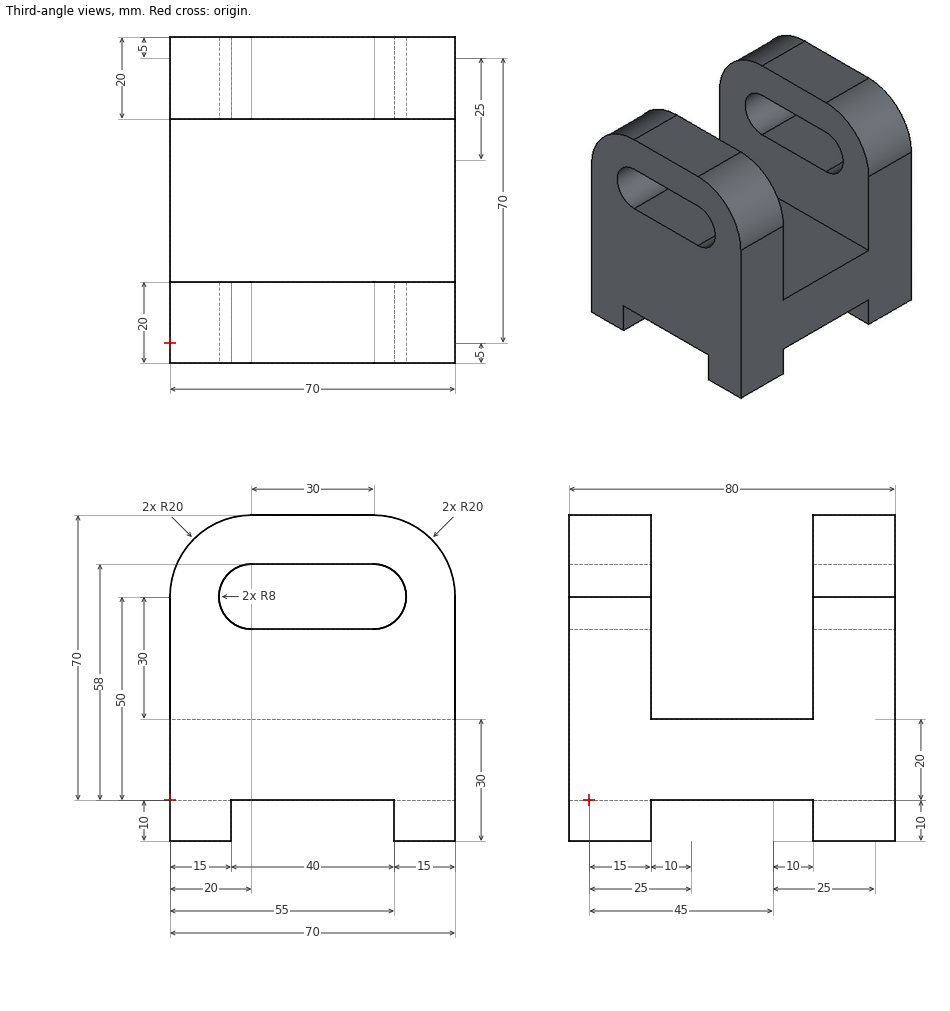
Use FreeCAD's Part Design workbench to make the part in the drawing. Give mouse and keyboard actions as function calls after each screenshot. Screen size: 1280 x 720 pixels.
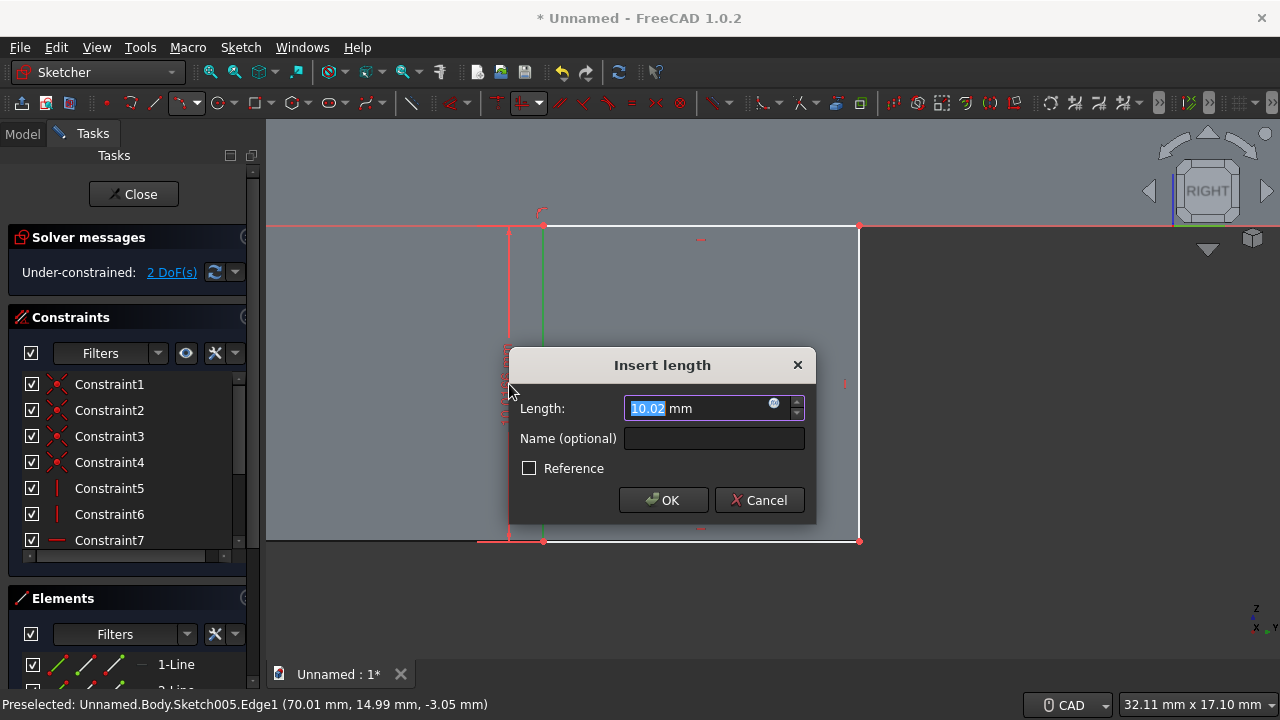
text(10)
key(Return)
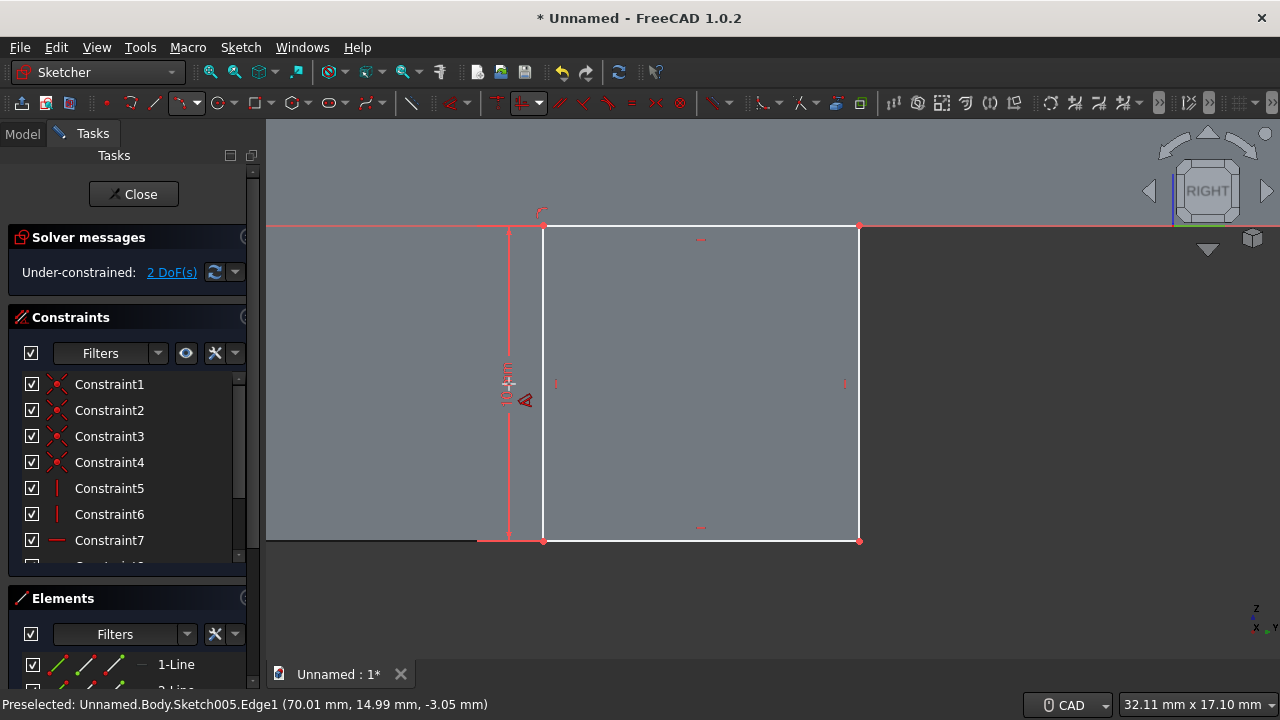
click(638, 541)
click(701, 575)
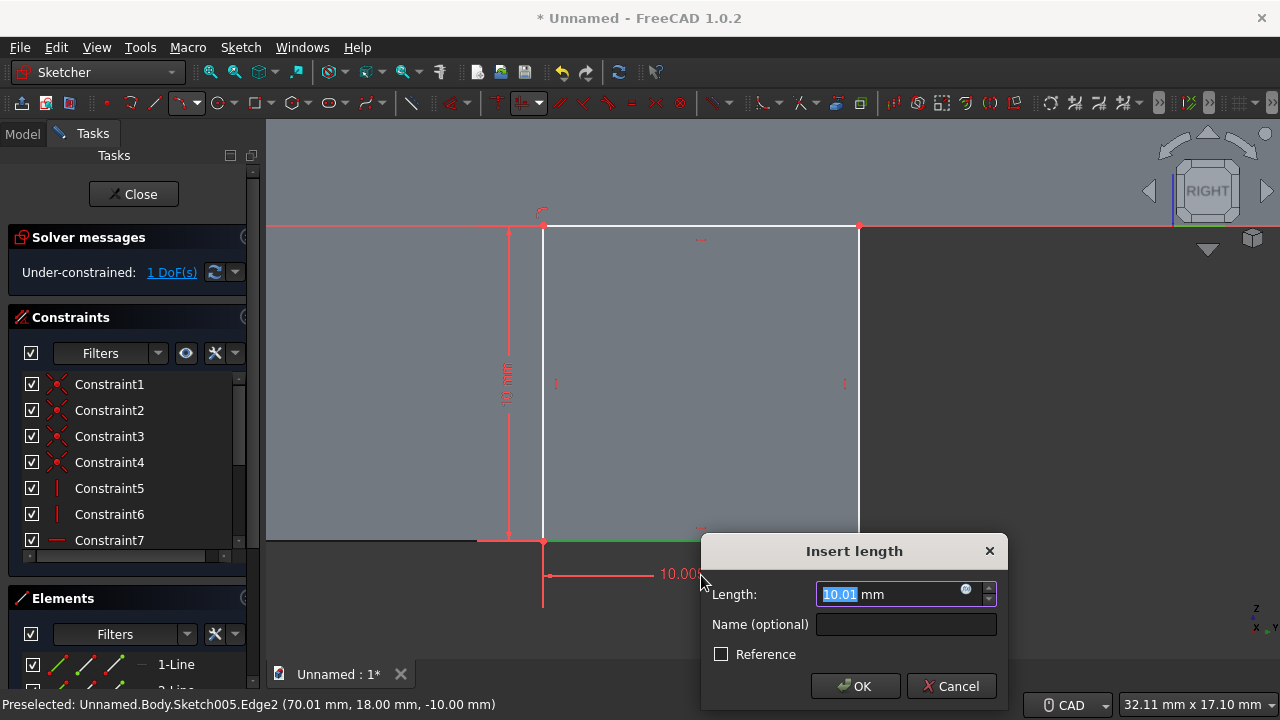
text(10)
key(Return)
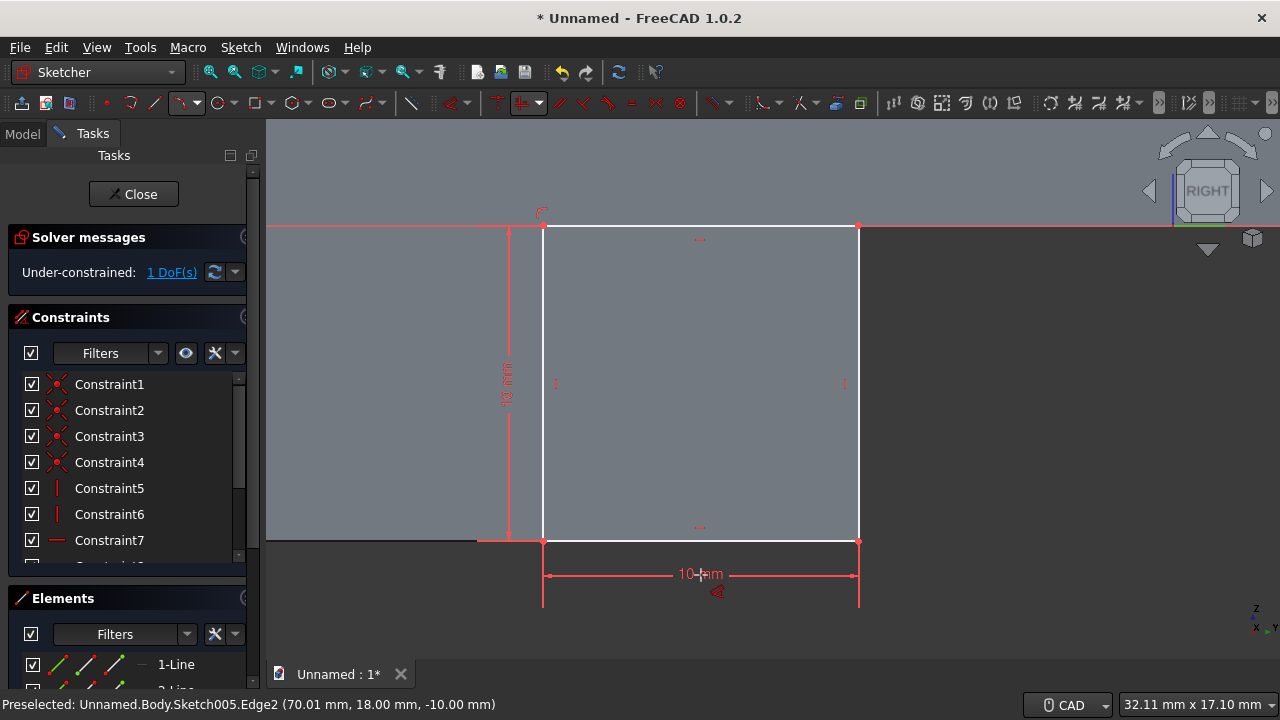
click(543, 226)
click(418, 192)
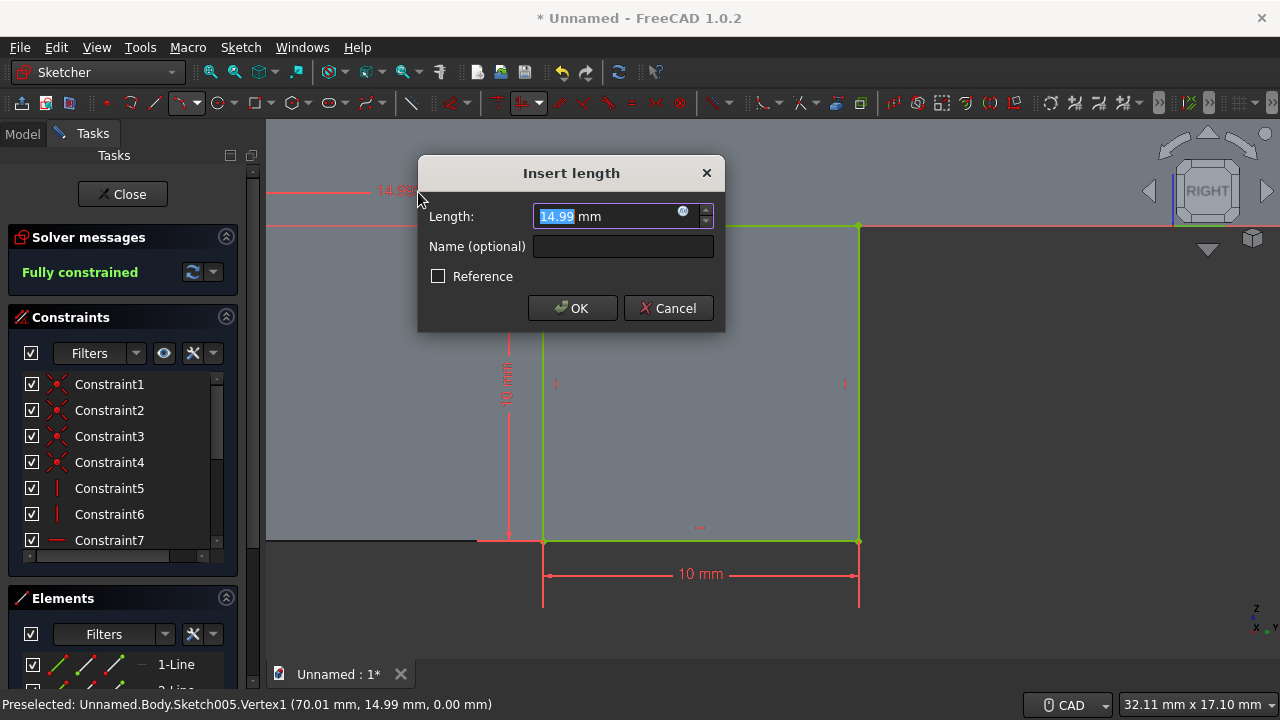
text(15)
key(Return)
key(Escape)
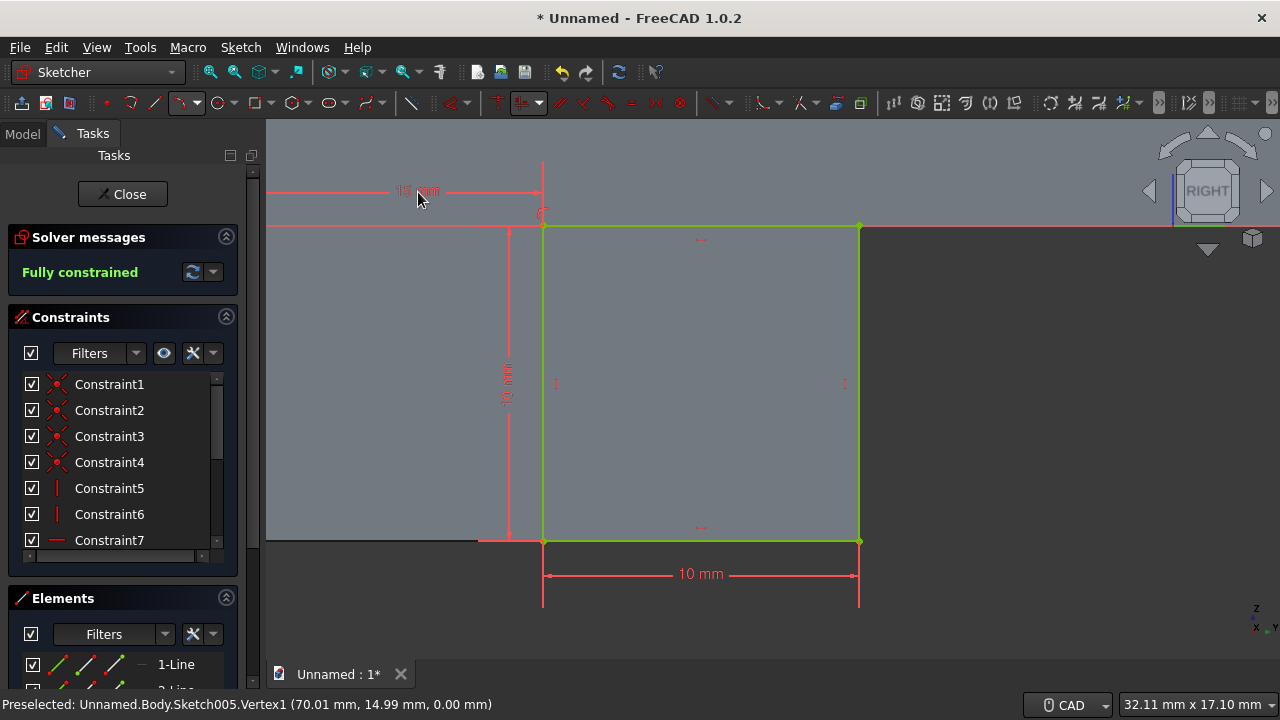
click(123, 194)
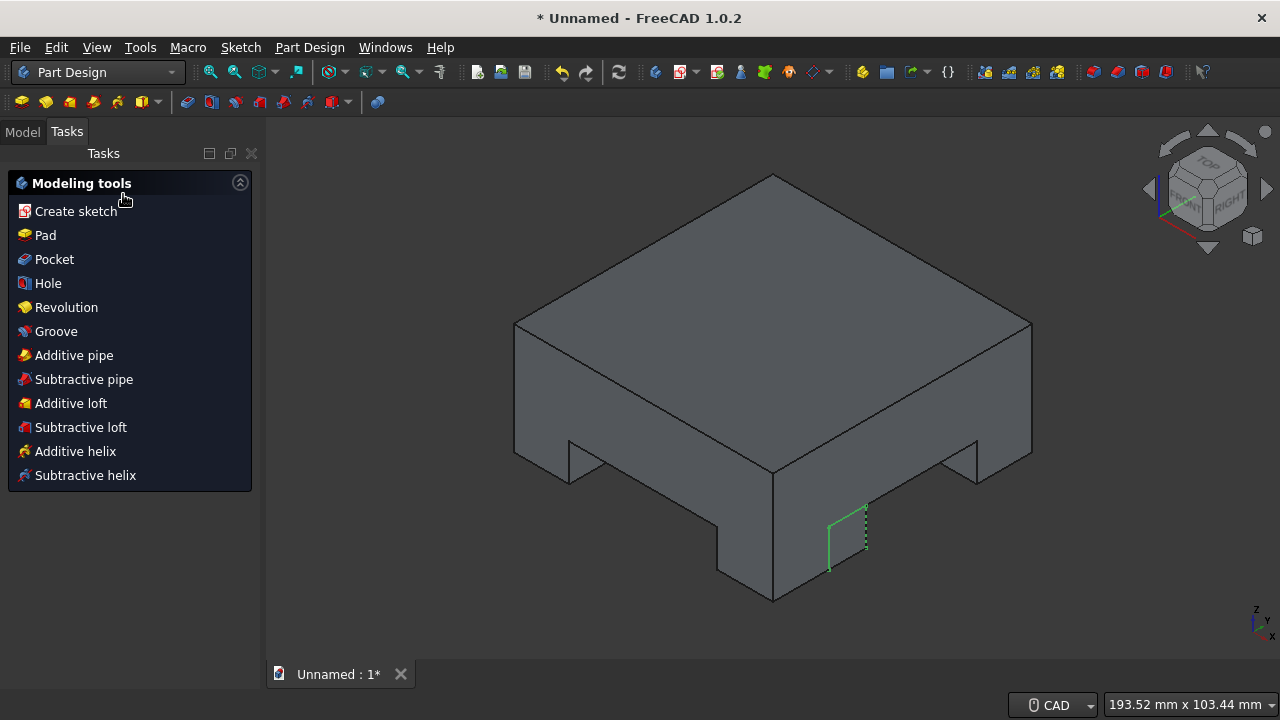
click(188, 102)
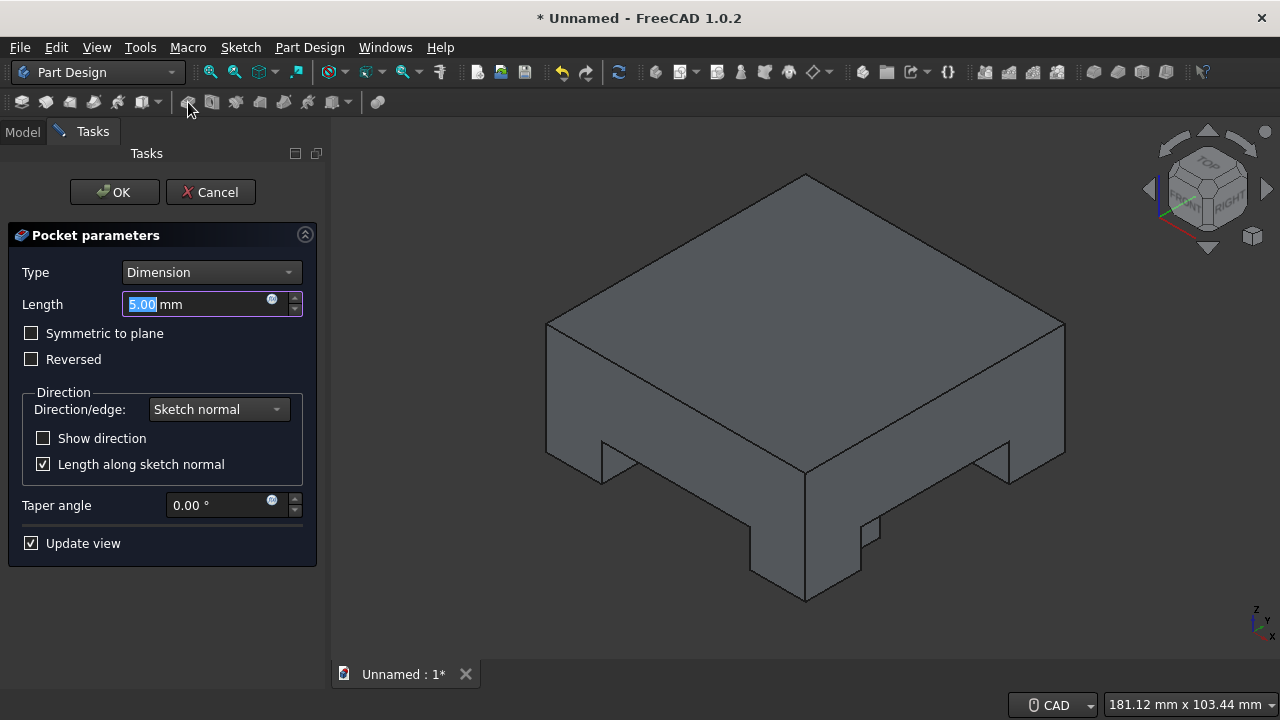
text(70)
key(Tab)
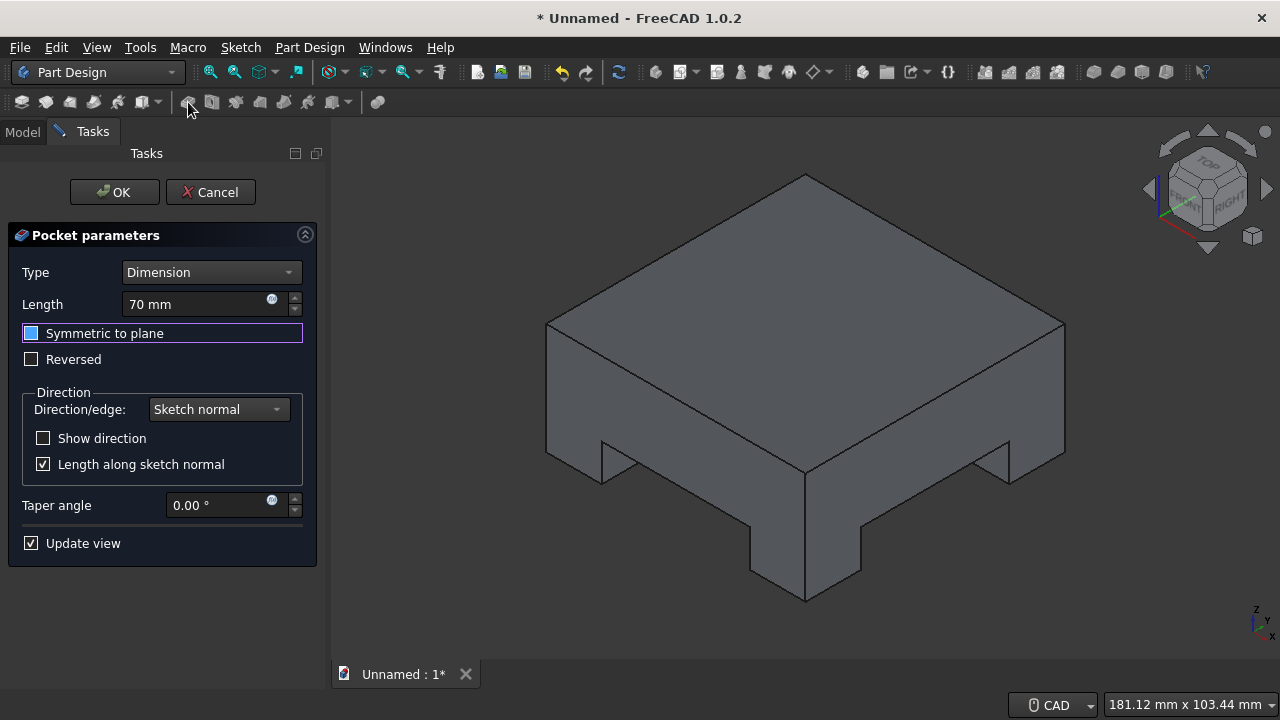
click(115, 192)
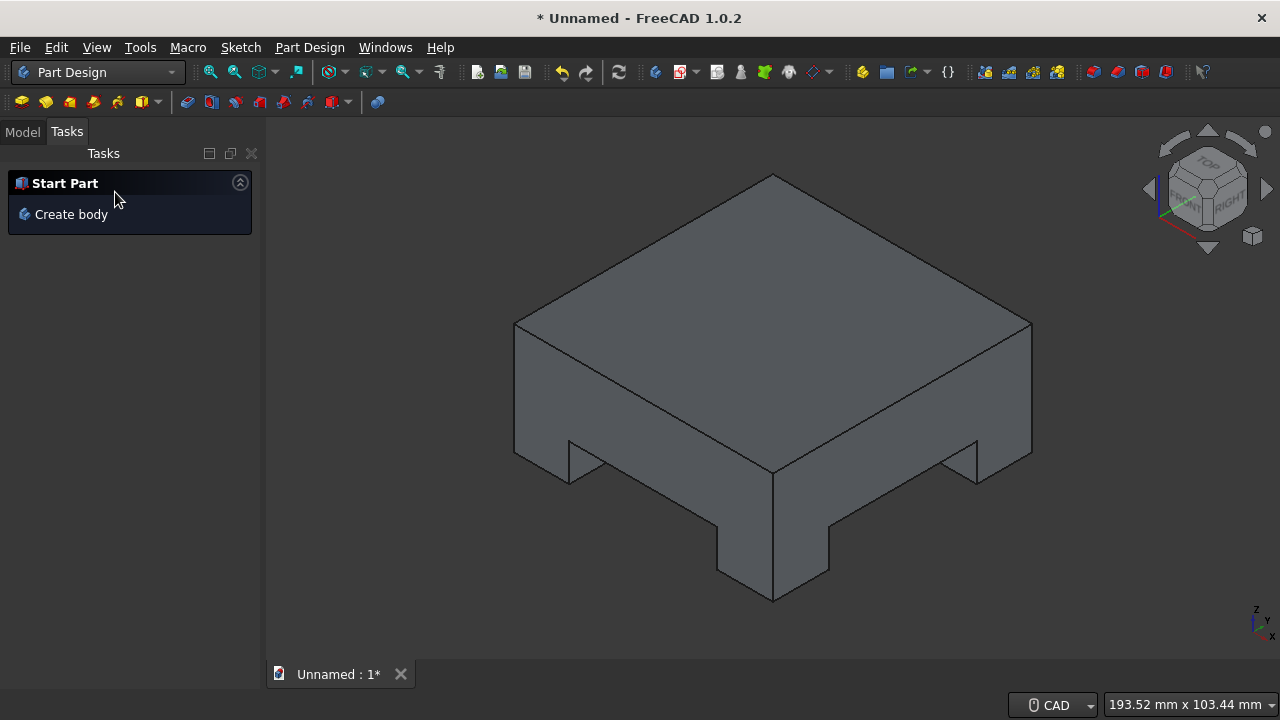
click(680, 72)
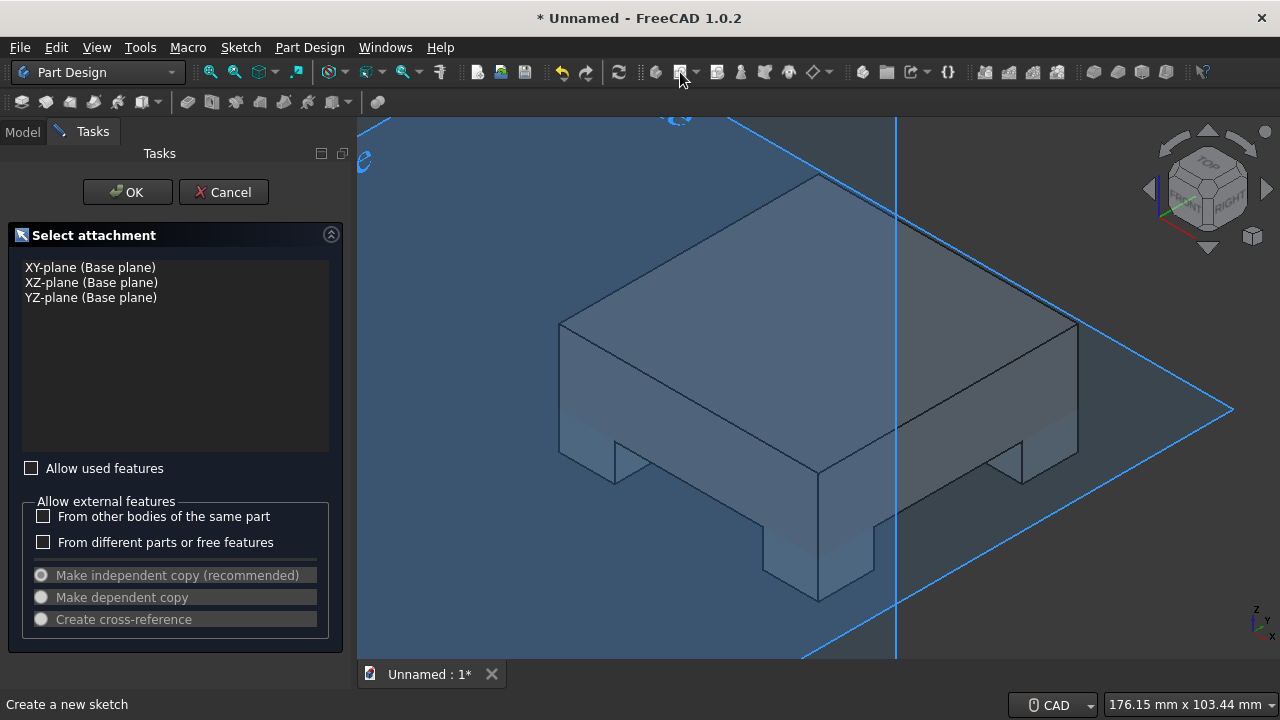
click(82, 282)